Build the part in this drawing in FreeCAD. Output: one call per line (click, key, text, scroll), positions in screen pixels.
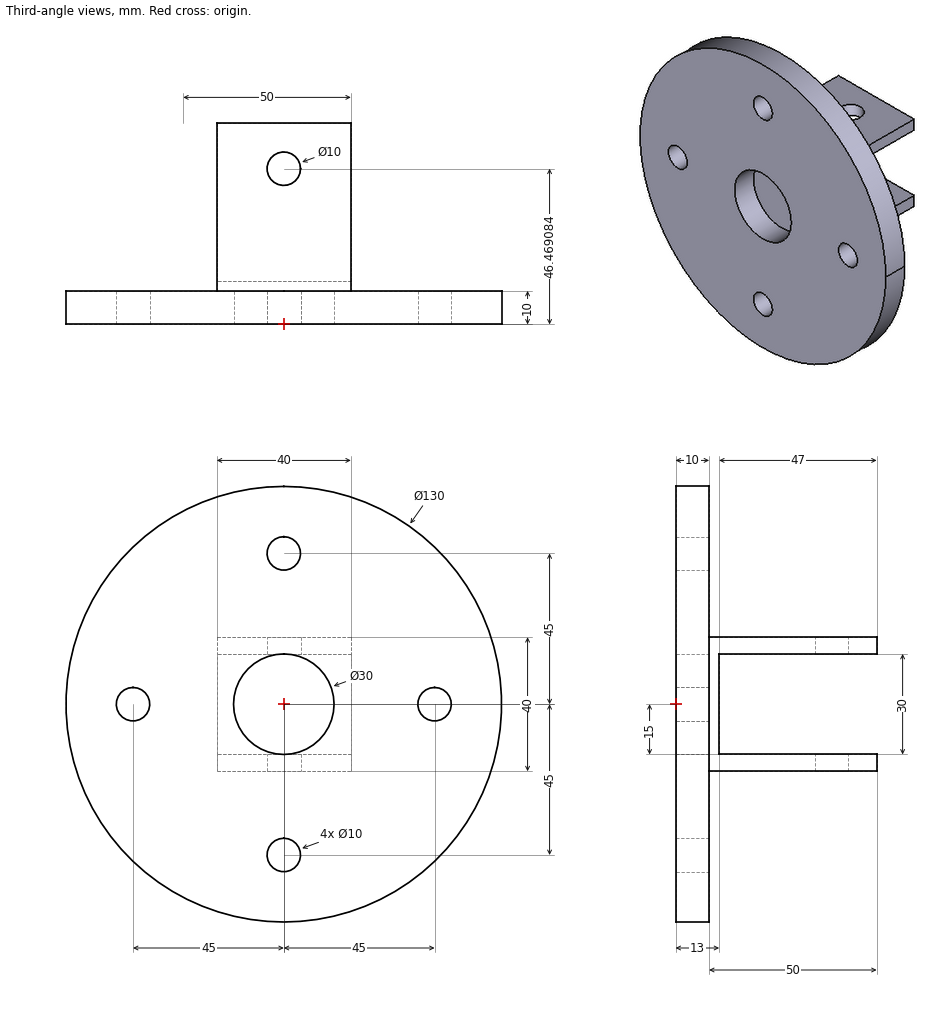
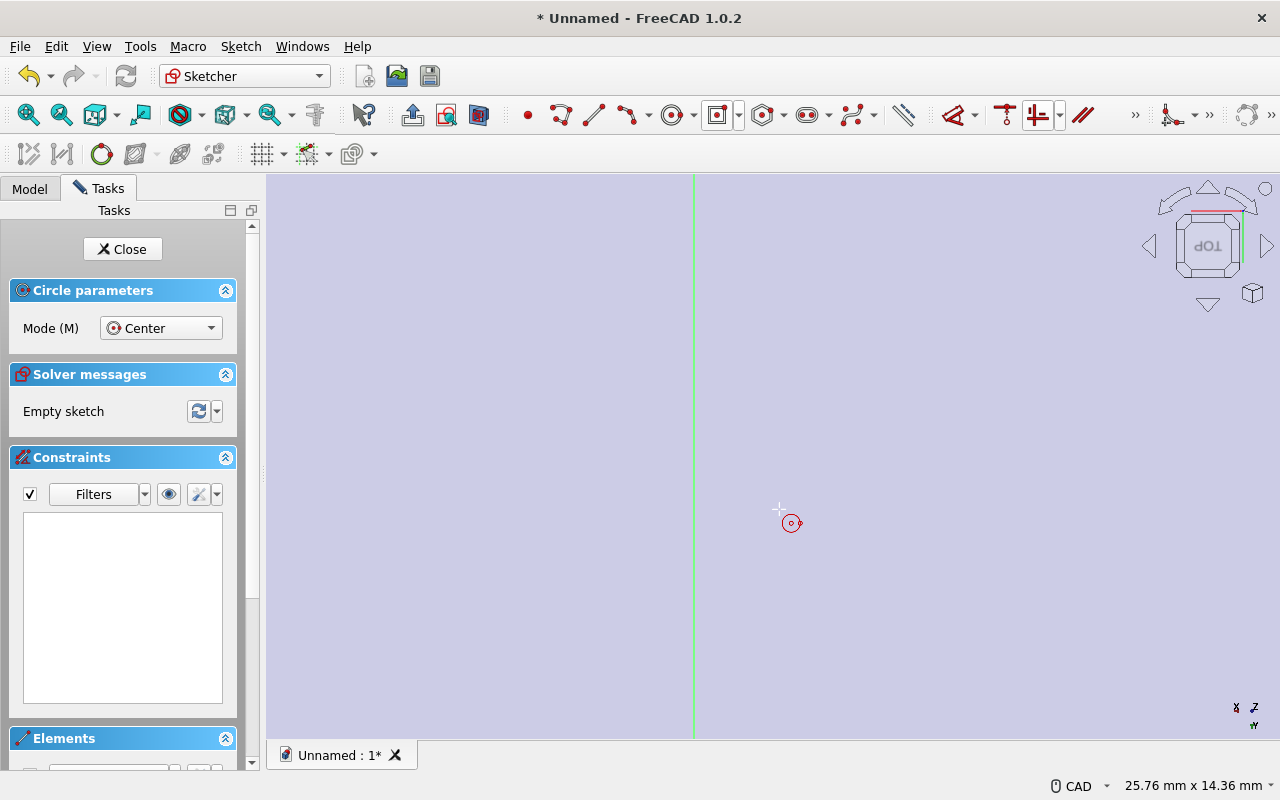
click(694, 443)
move(833, 304)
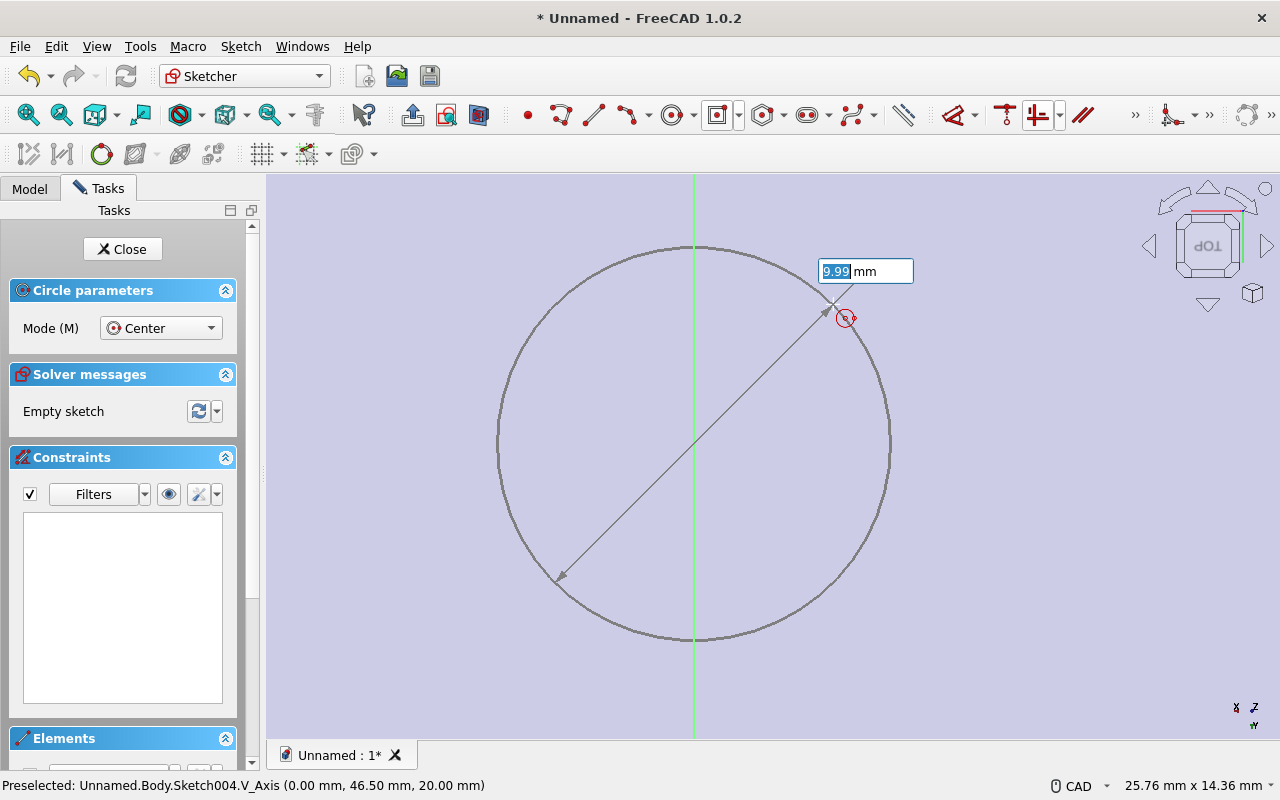
text(10)
key(Return)
key(Escape)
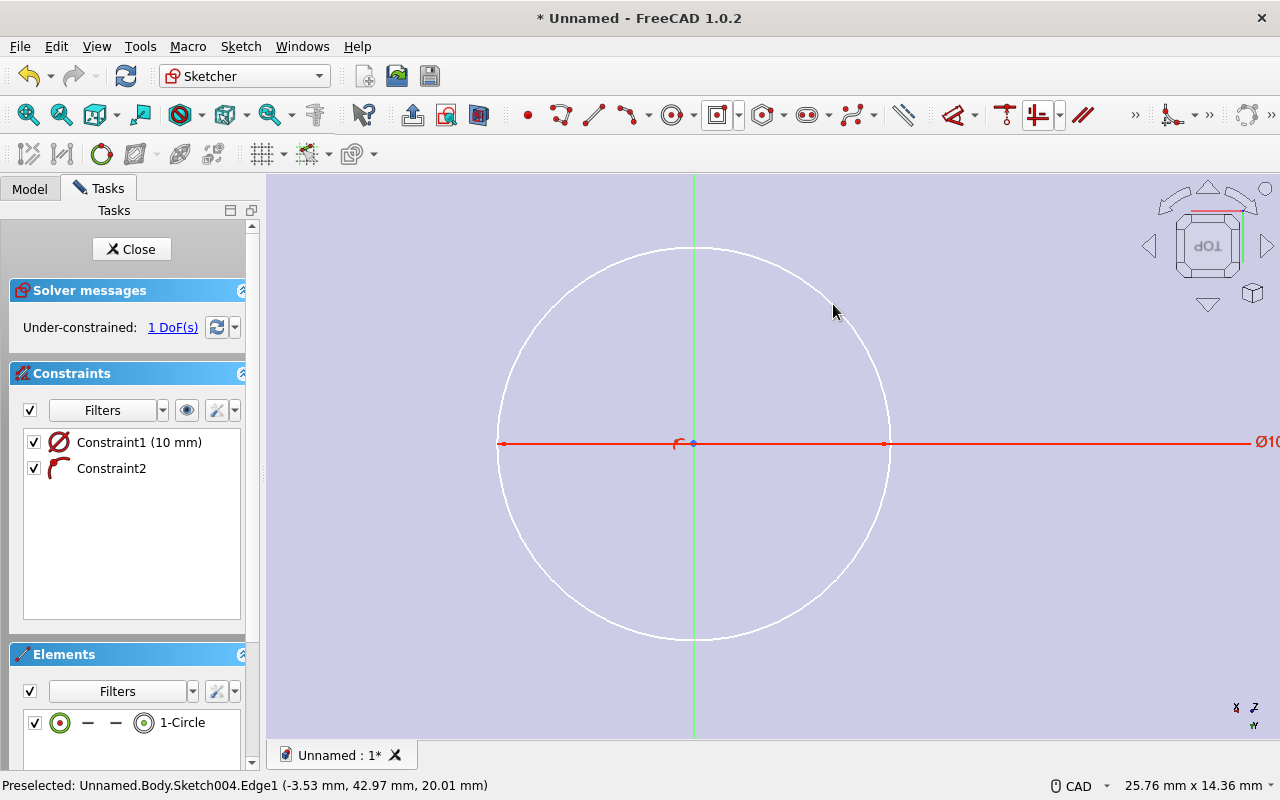
key(d)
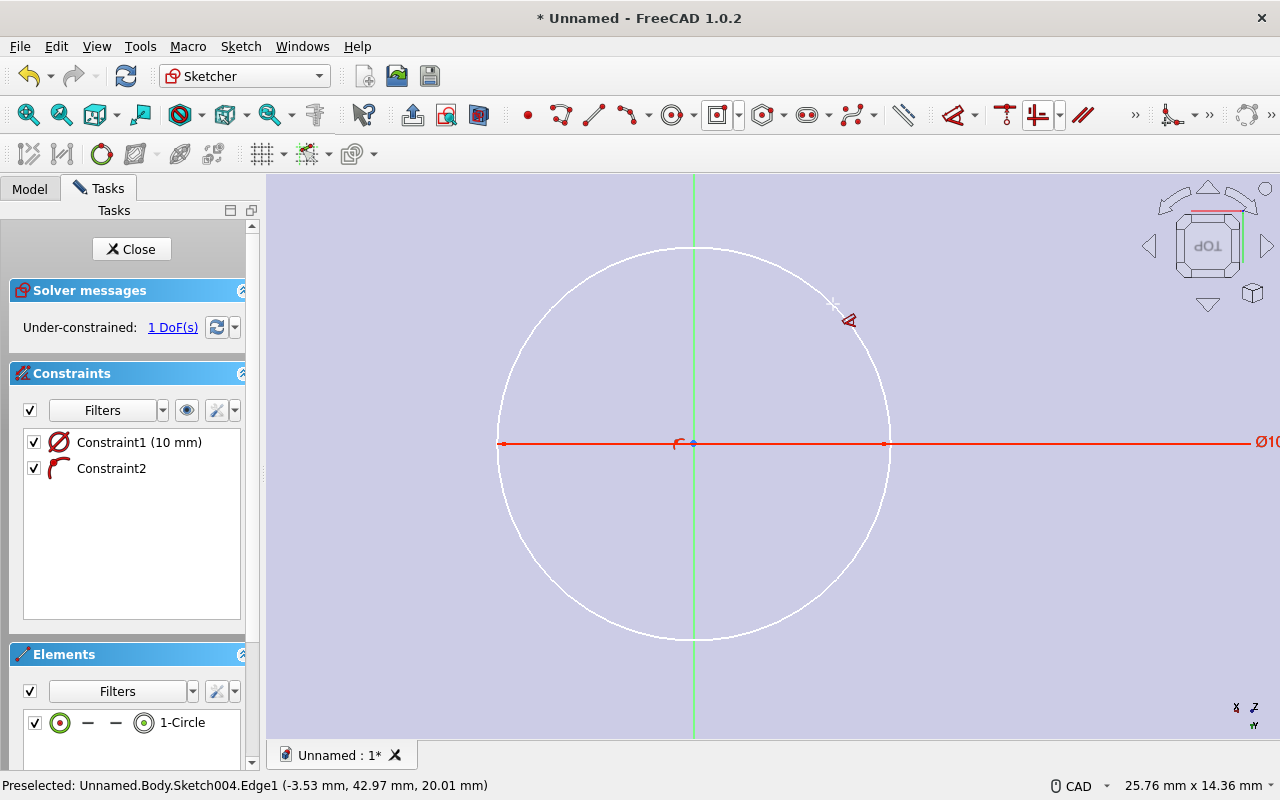
click(694, 444)
click(728, 323)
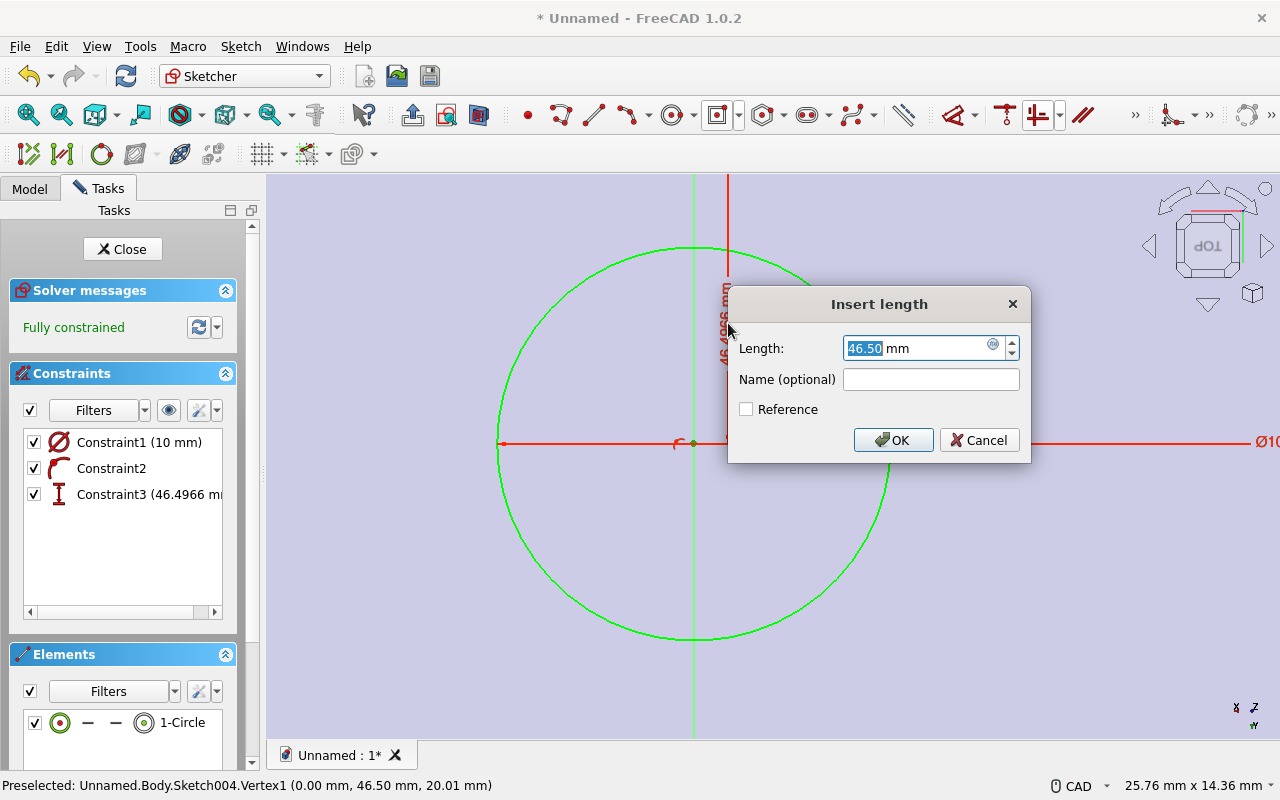
text(46.469084)
key(Return)
key(Escape)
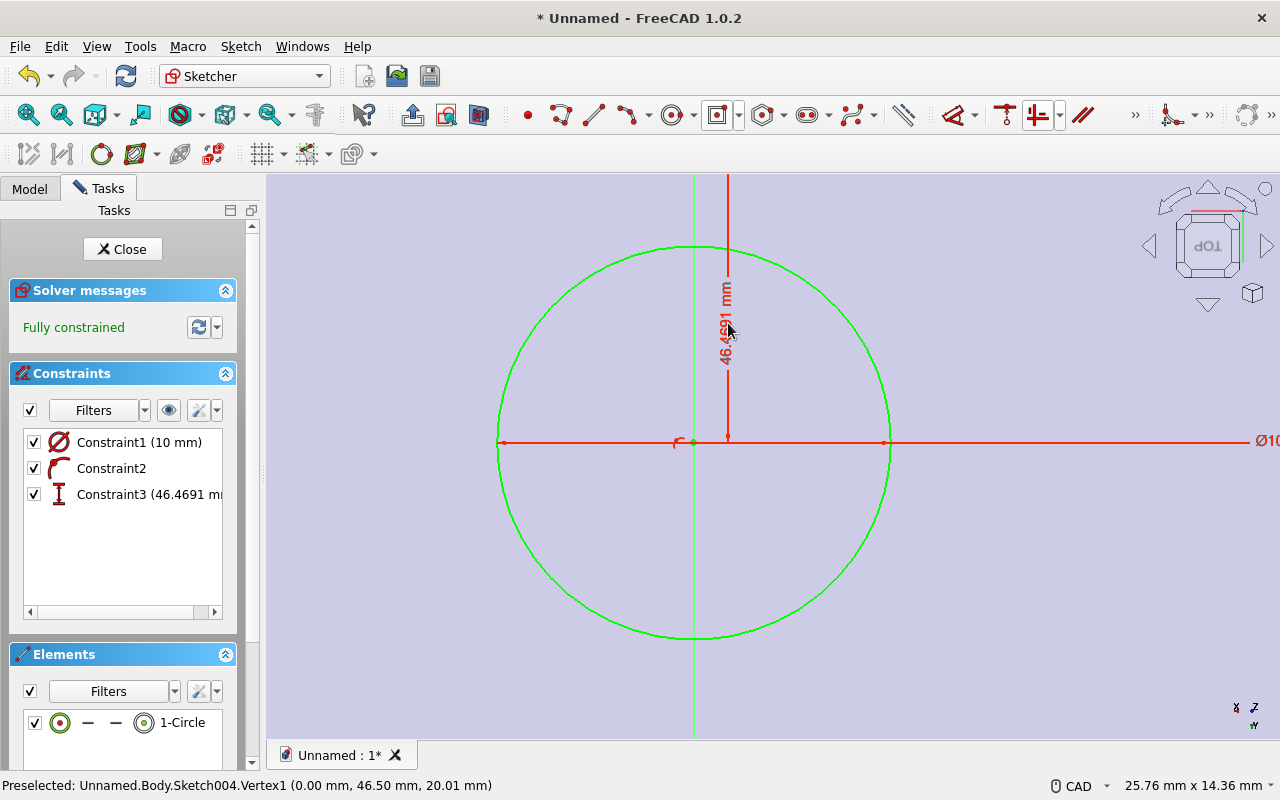
click(123, 249)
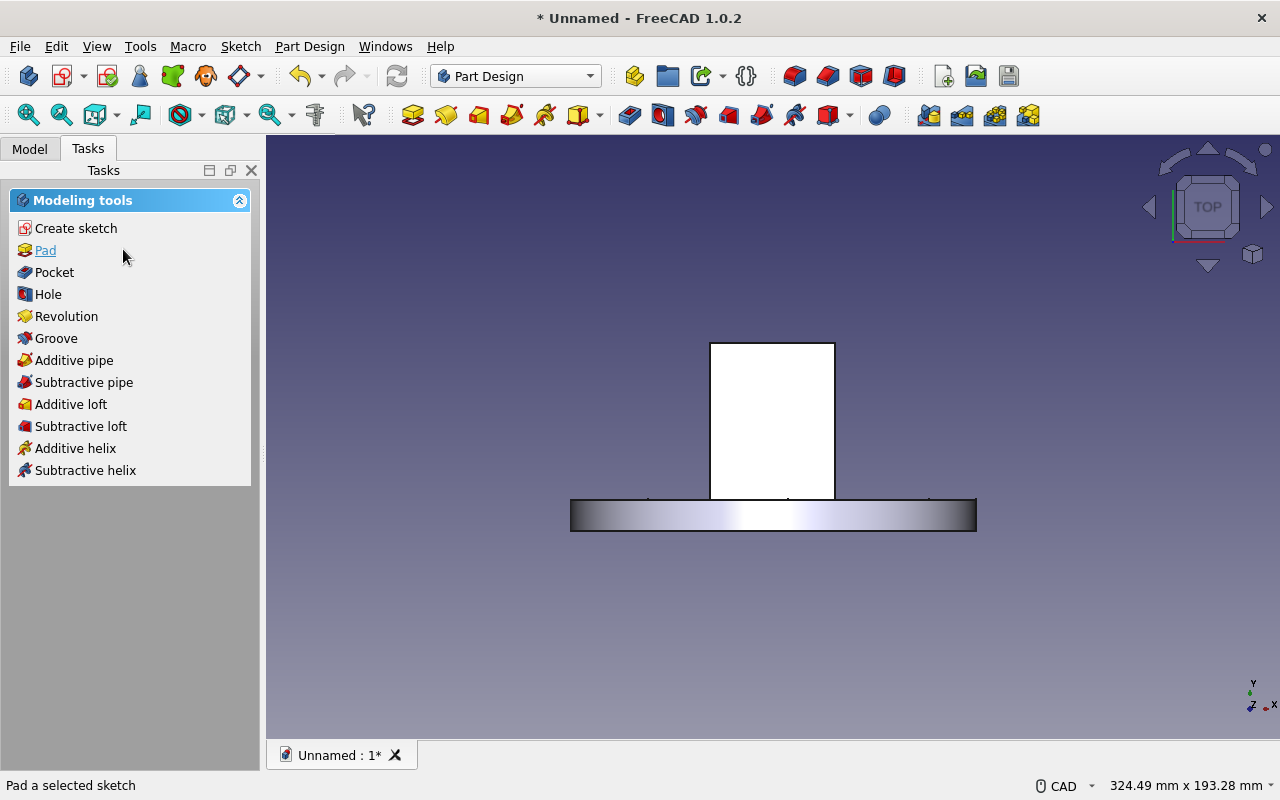
click(630, 116)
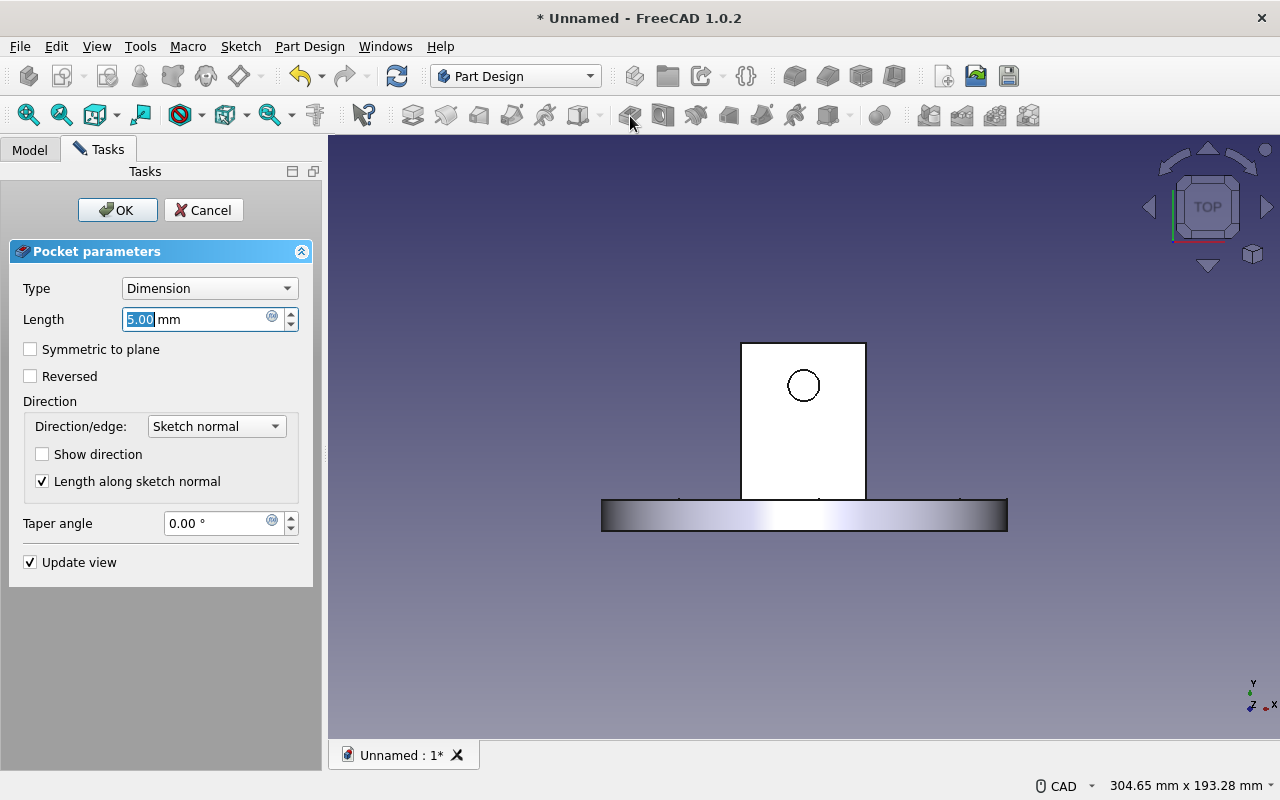
click(210, 288)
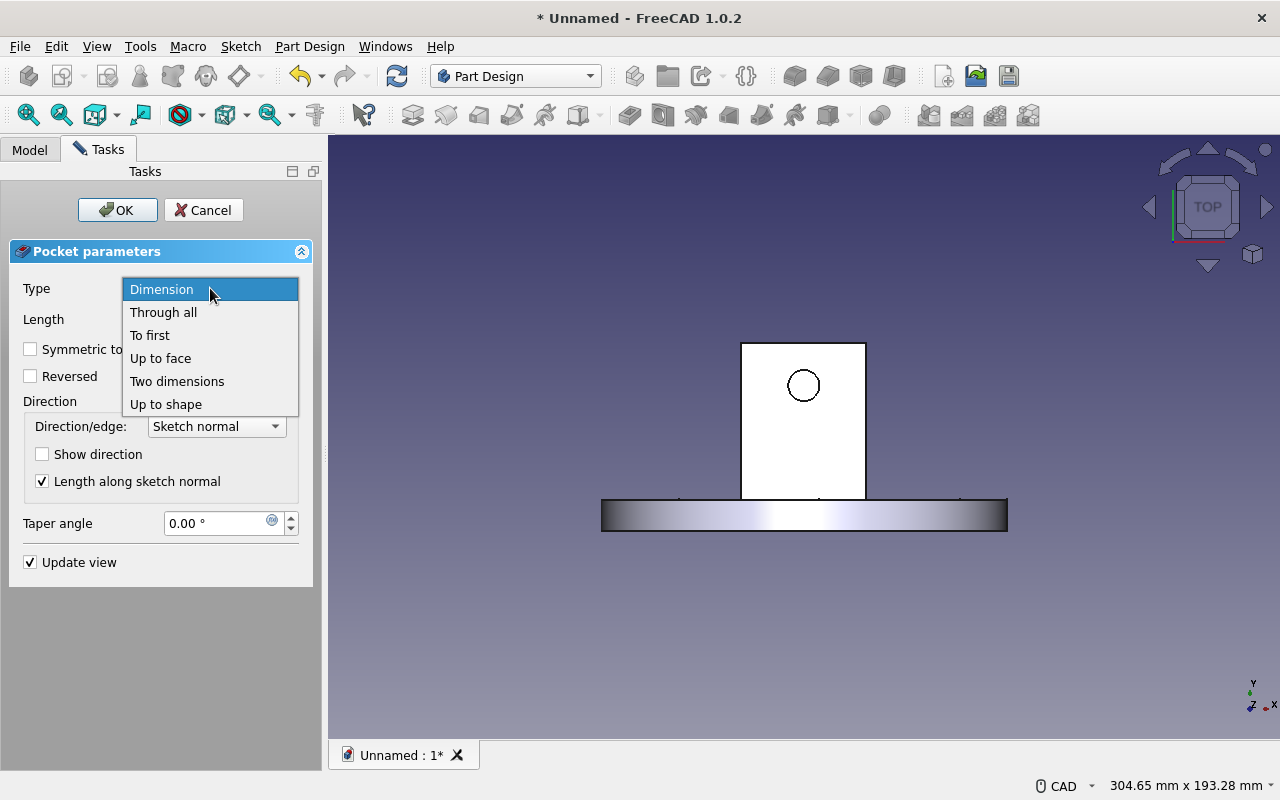
click(208, 312)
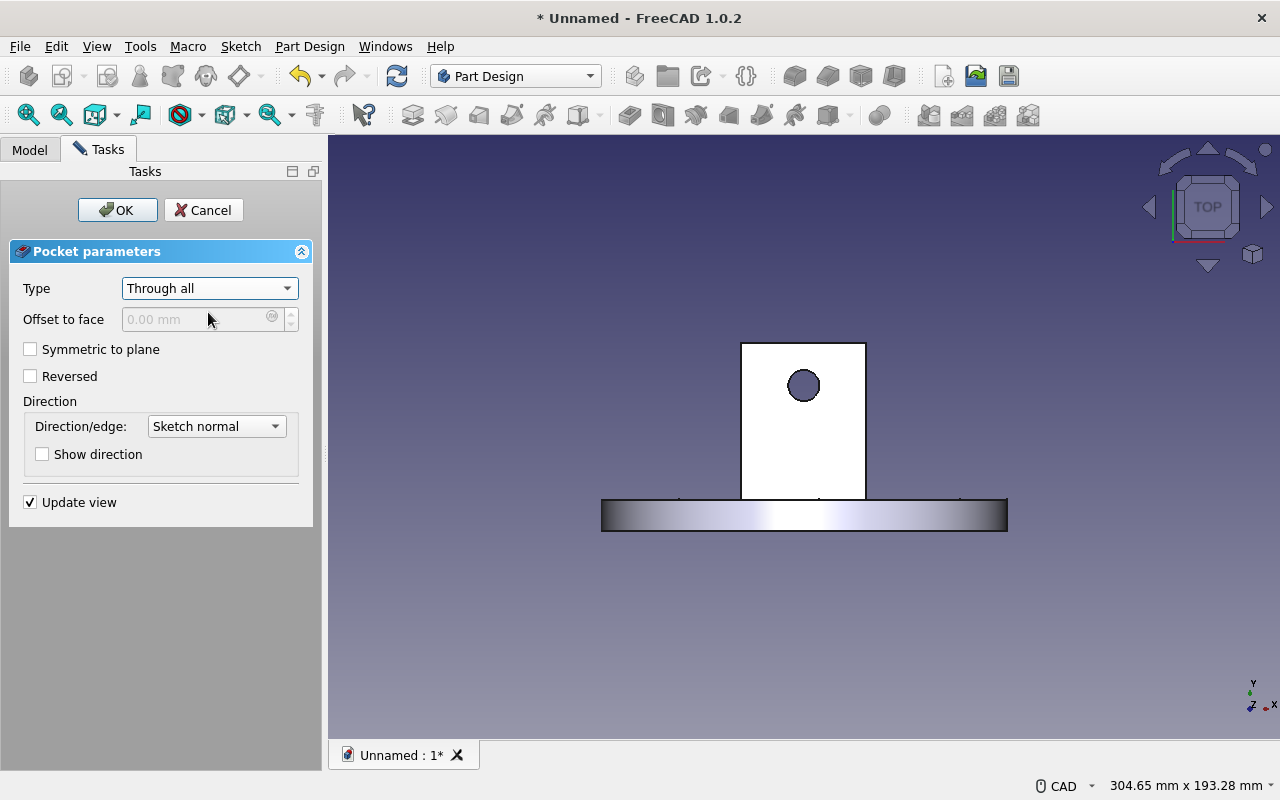
click(118, 210)